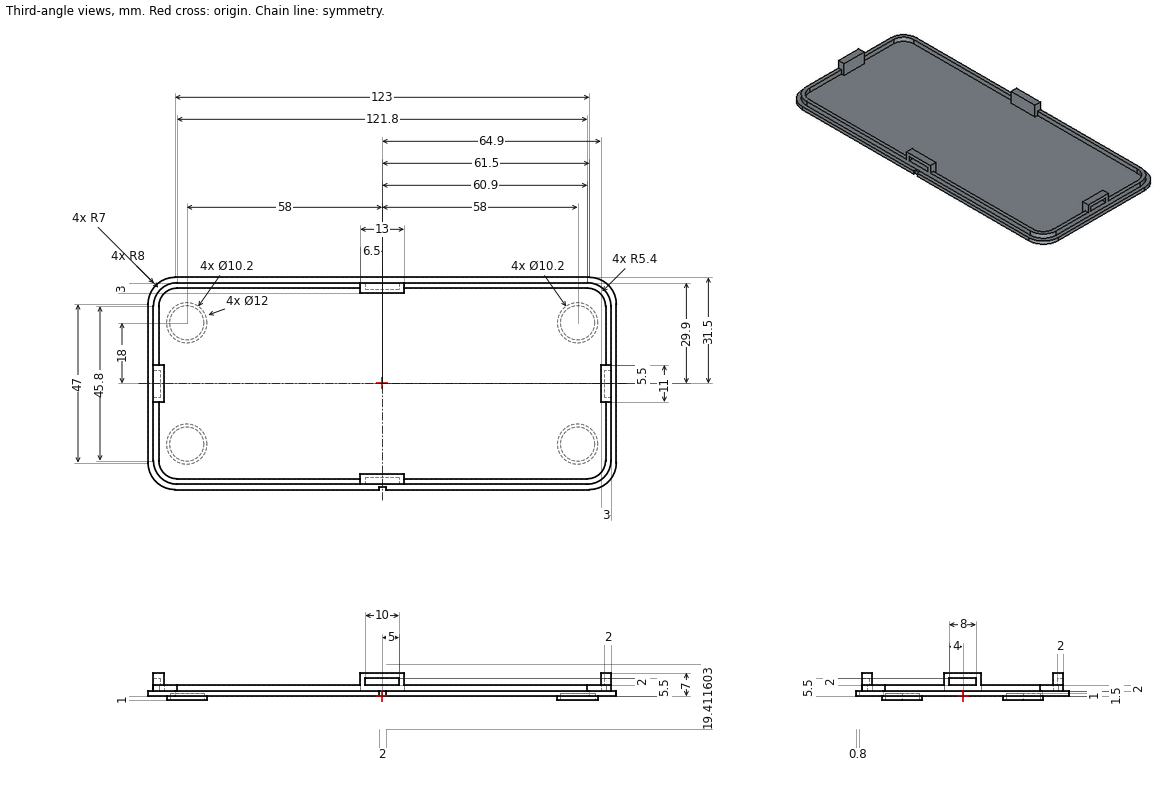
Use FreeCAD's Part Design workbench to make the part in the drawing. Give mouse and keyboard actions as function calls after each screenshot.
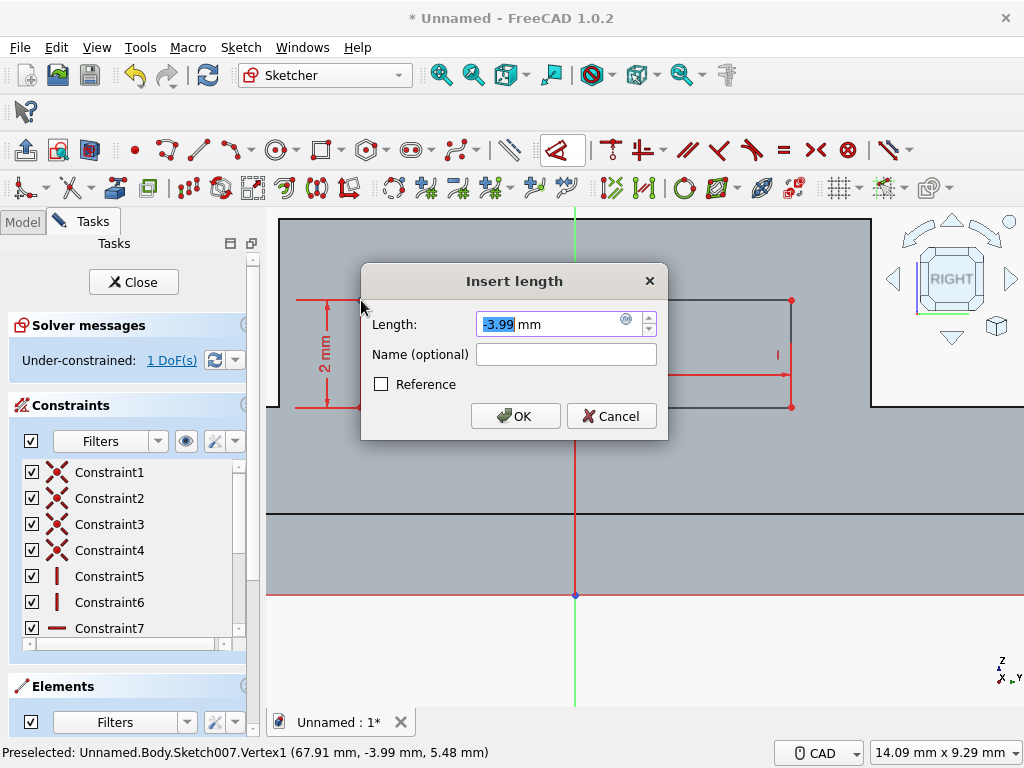
text(-4)
key(Return)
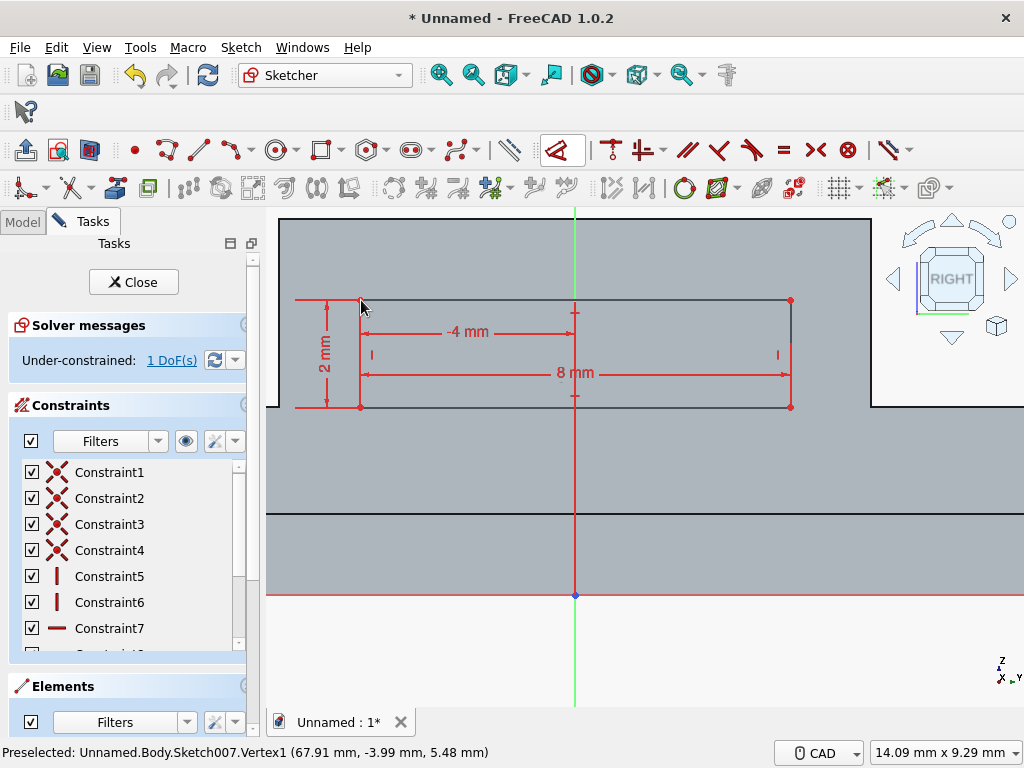
click(360, 300)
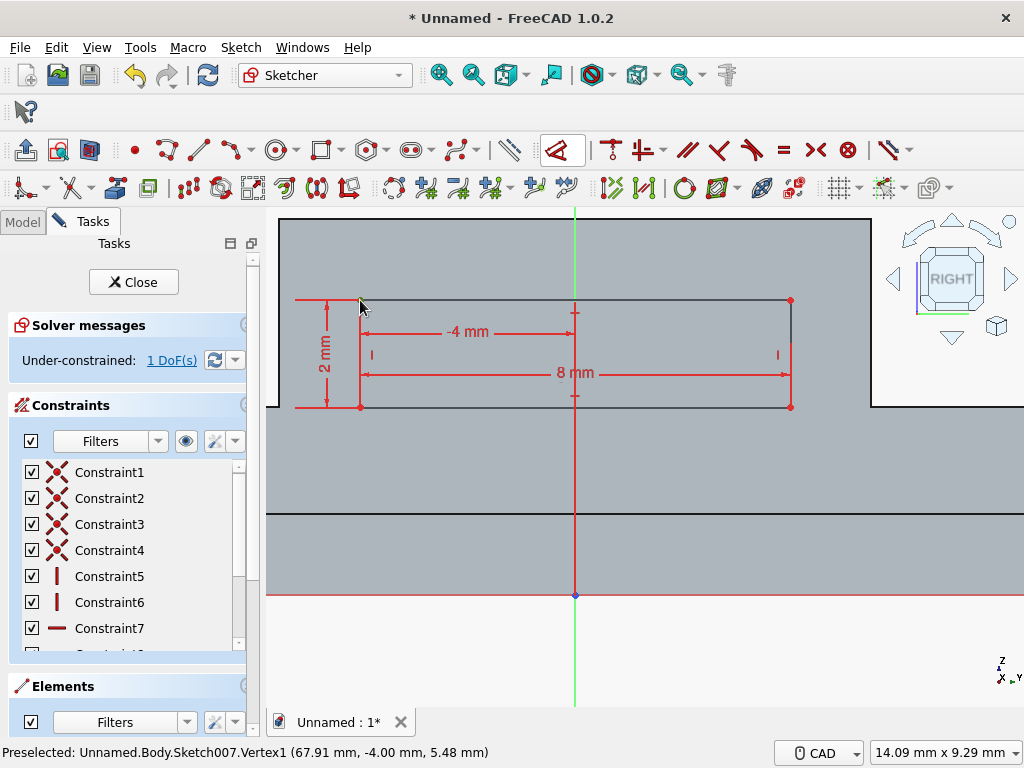
key(i)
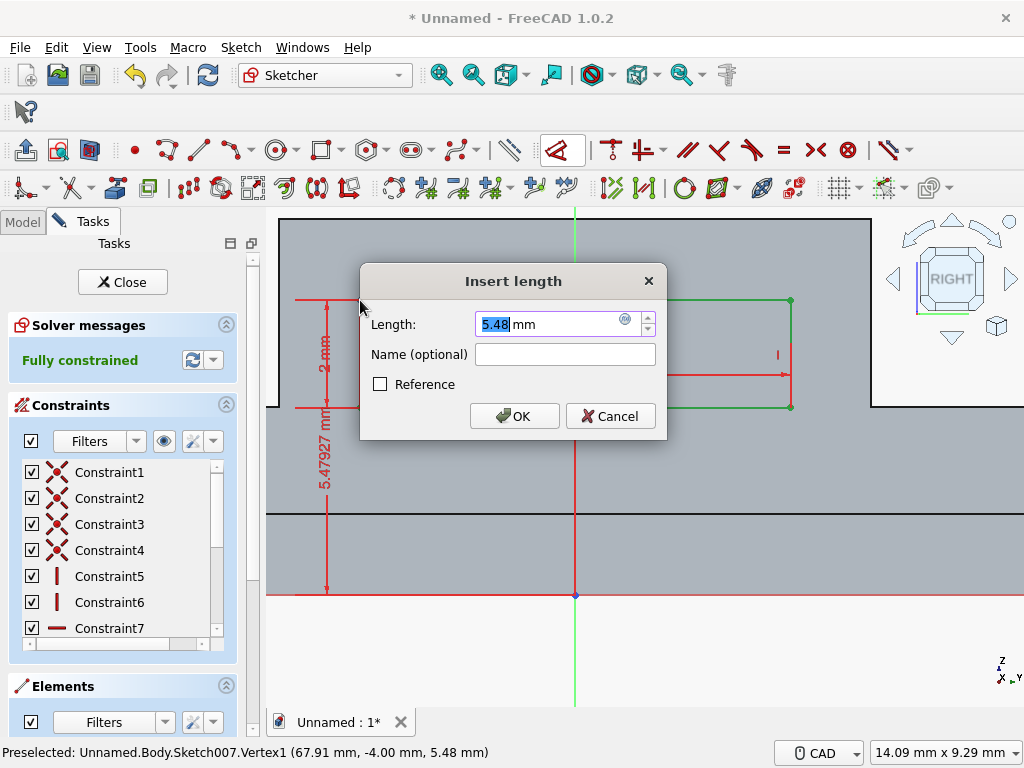
text(5.5)
key(Return)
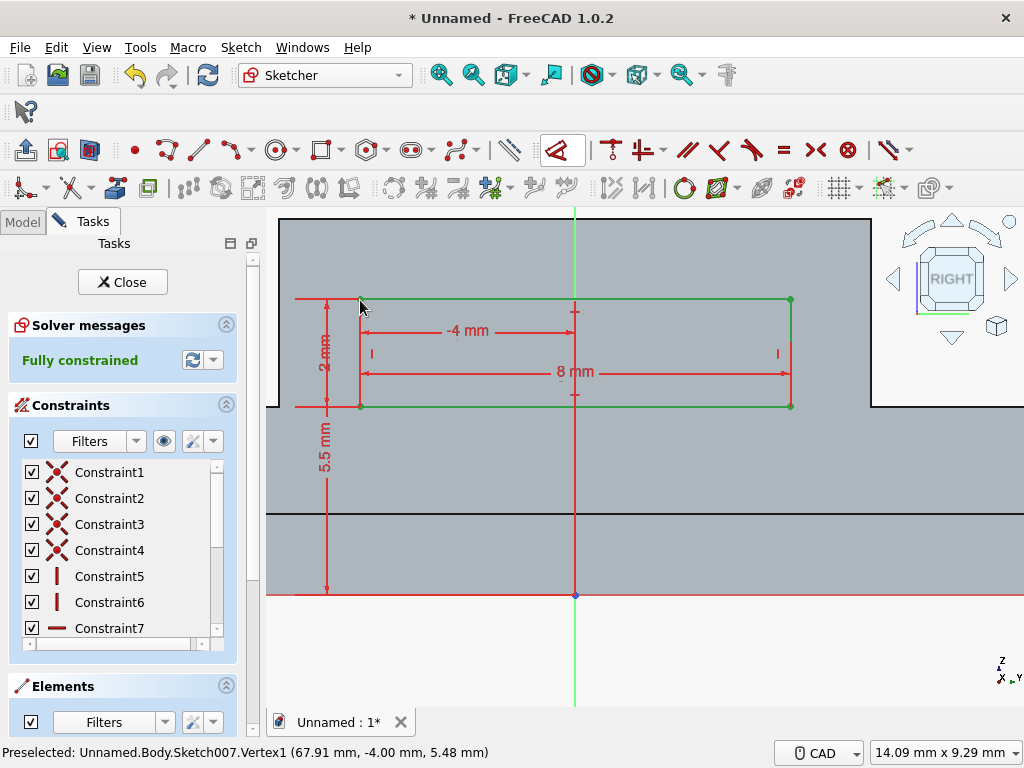
click(123, 282)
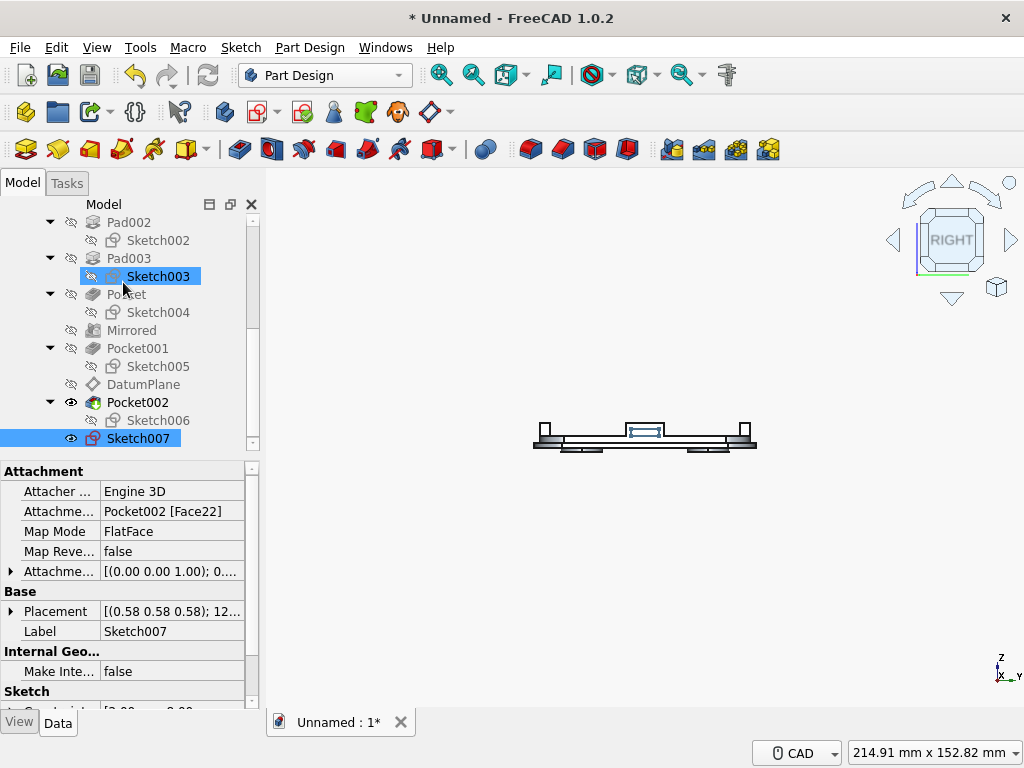
click(240, 150)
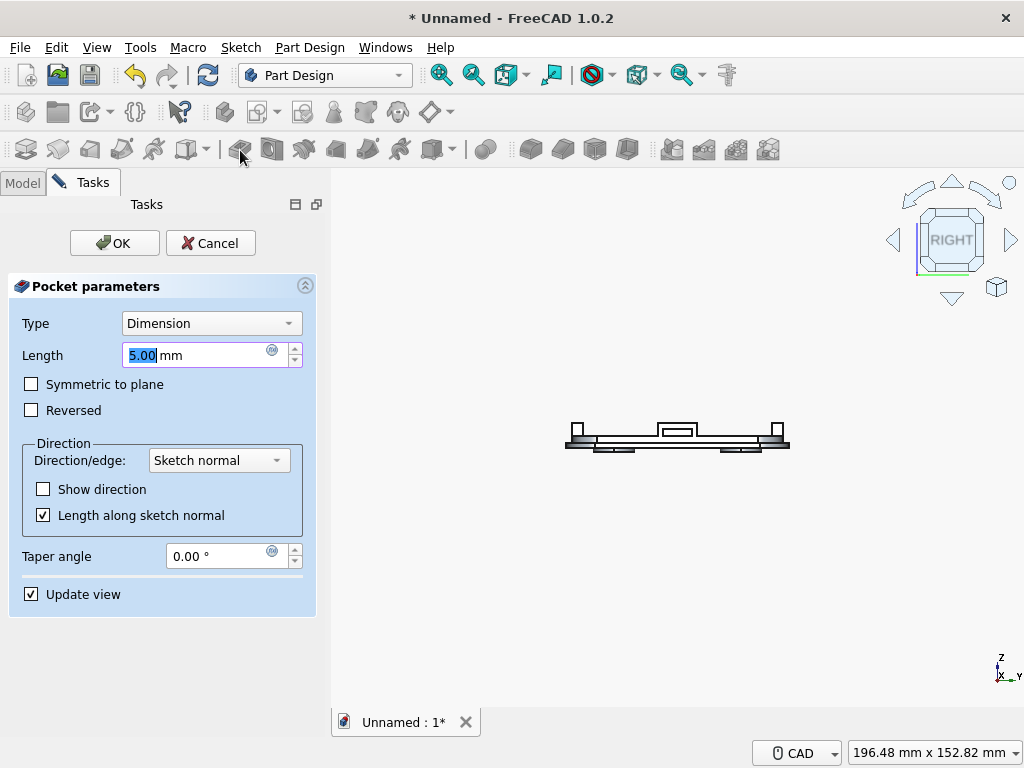
text(2)
key(Tab)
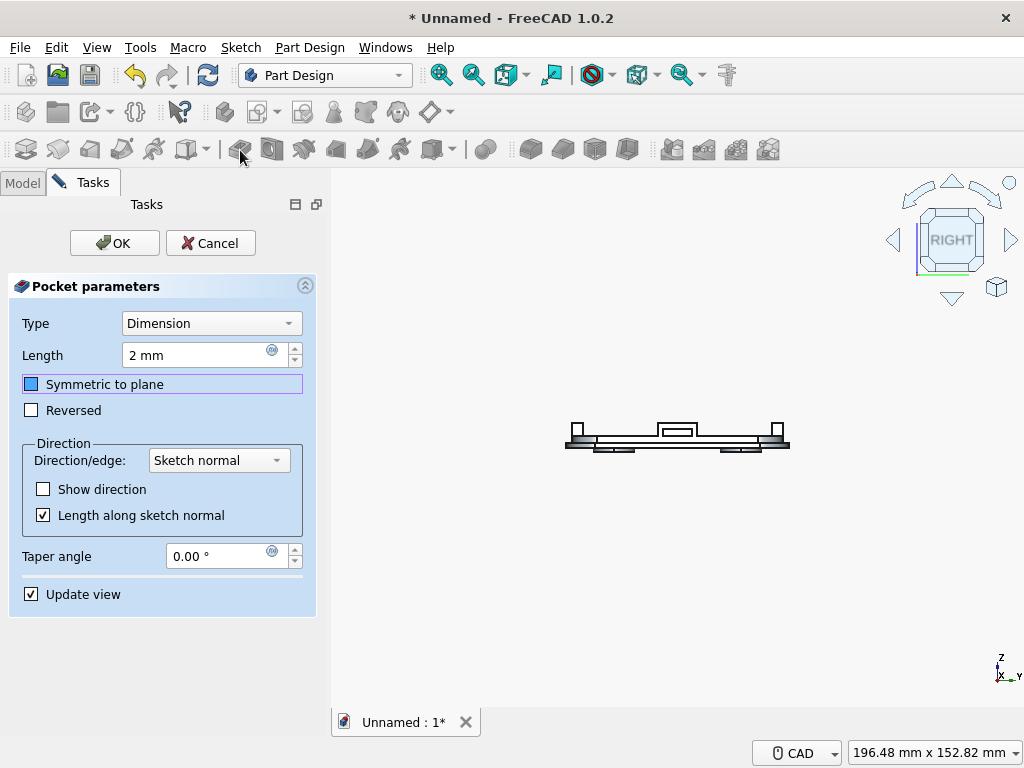
click(115, 243)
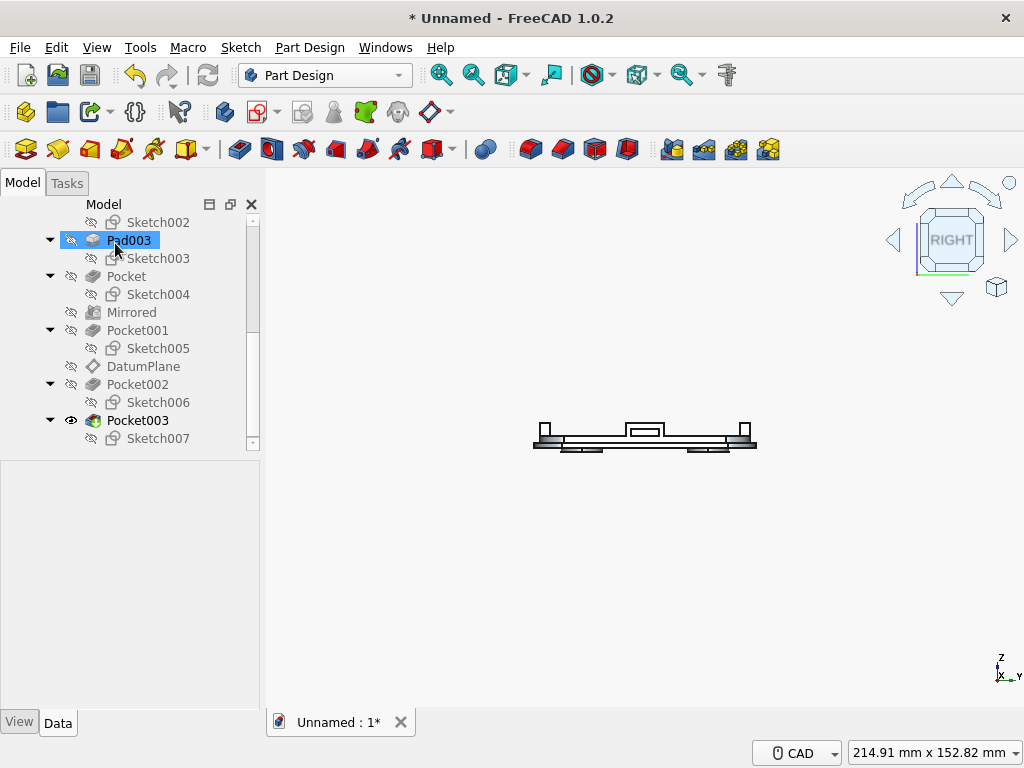
key(v)
key(f)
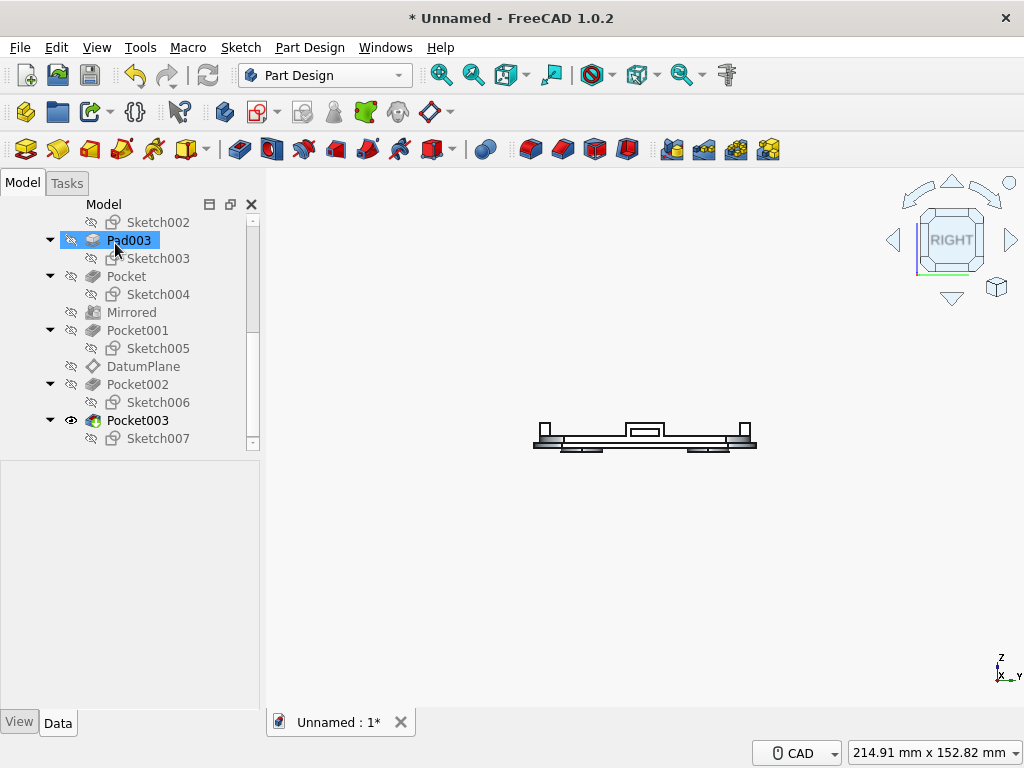
click(116, 420)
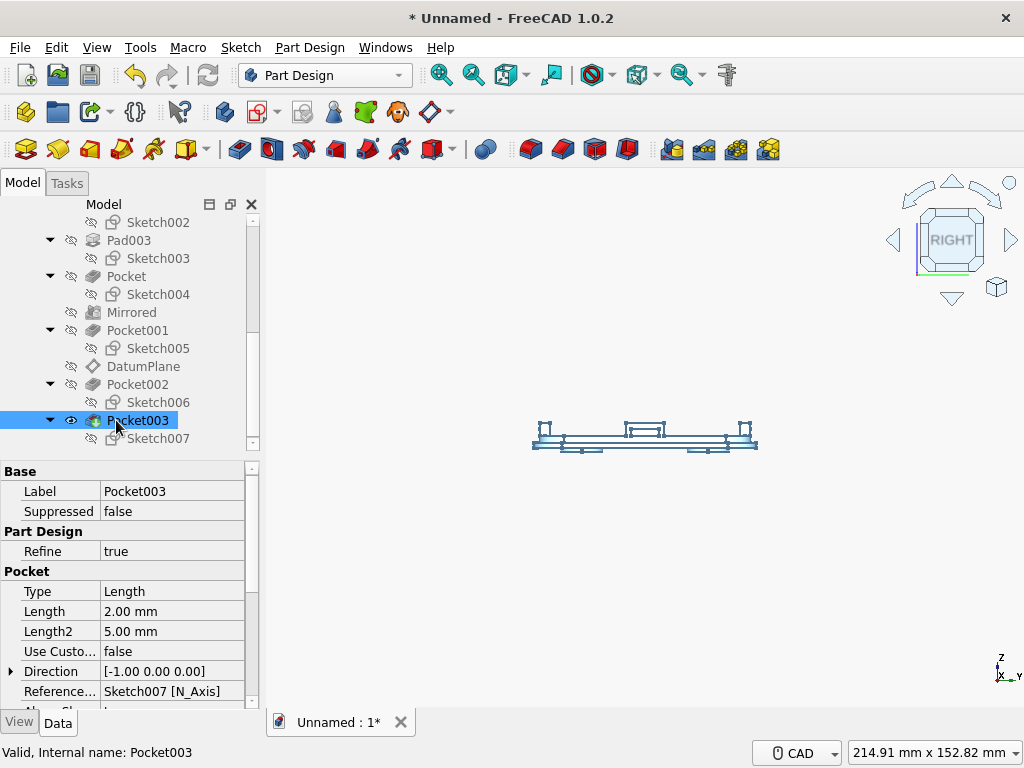
click(672, 150)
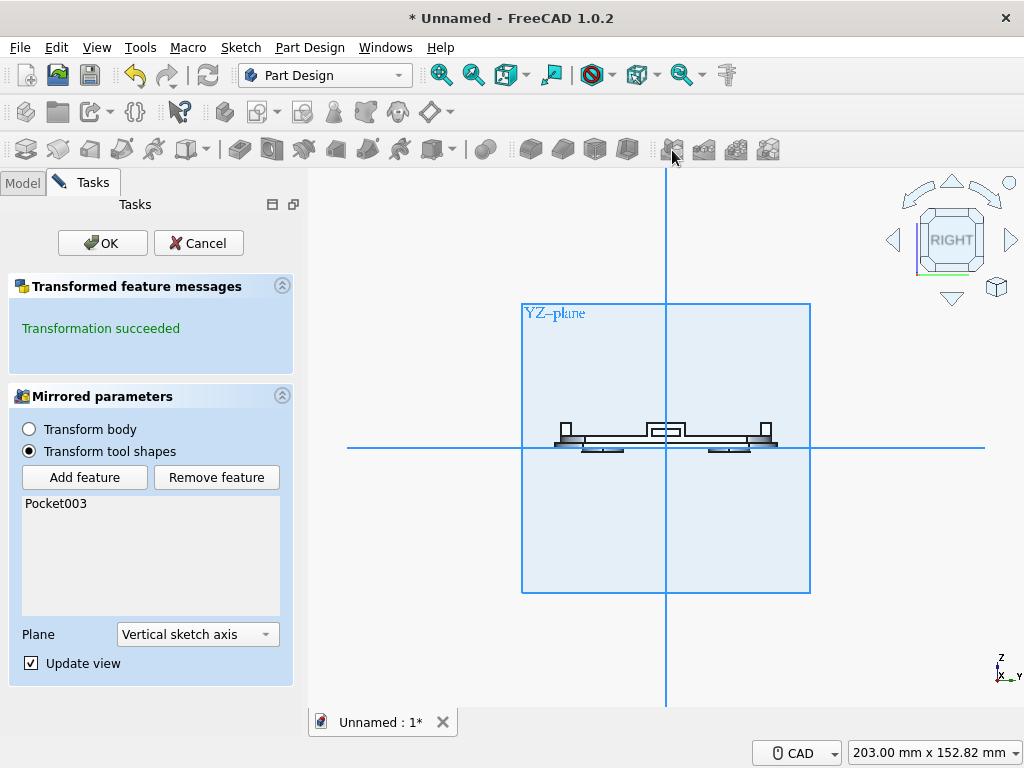
click(198, 634)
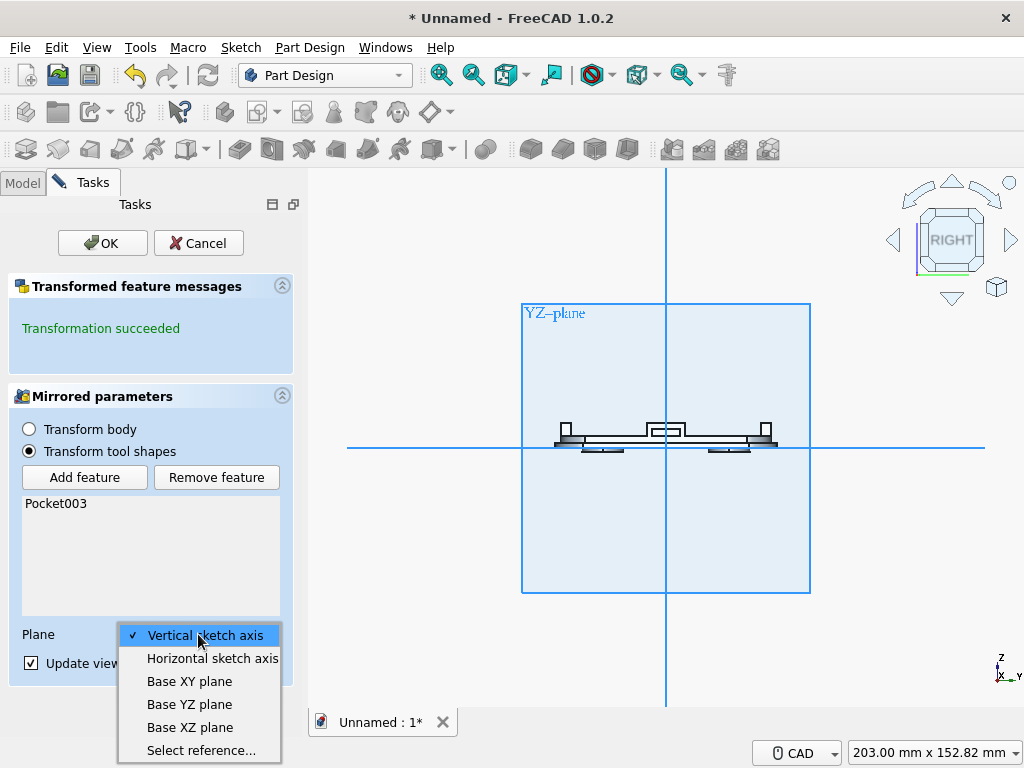
click(198, 704)